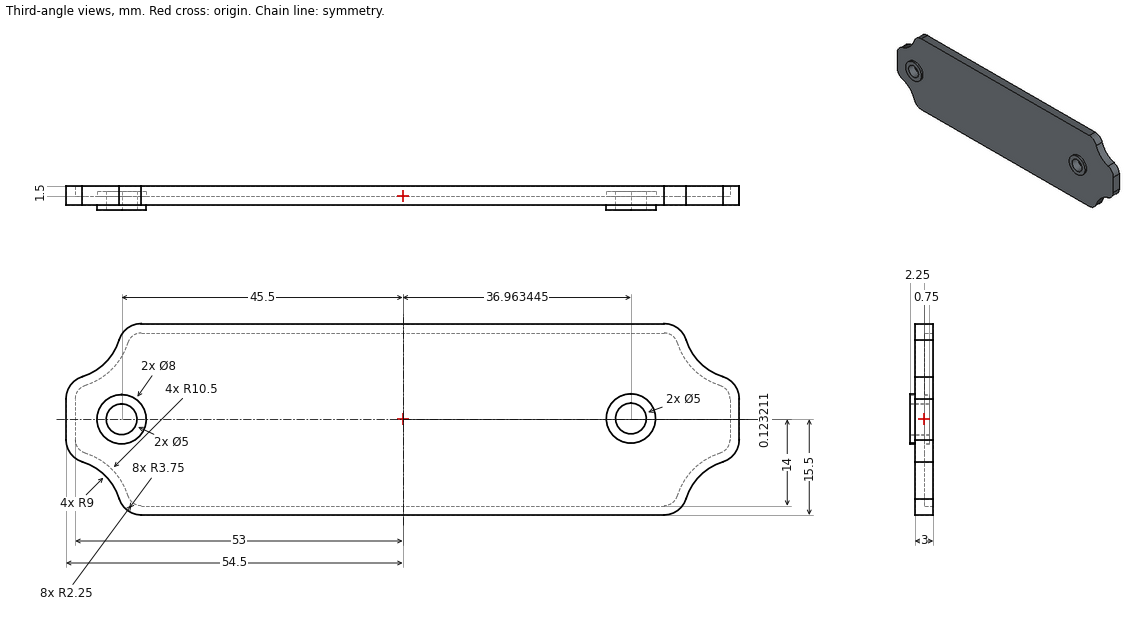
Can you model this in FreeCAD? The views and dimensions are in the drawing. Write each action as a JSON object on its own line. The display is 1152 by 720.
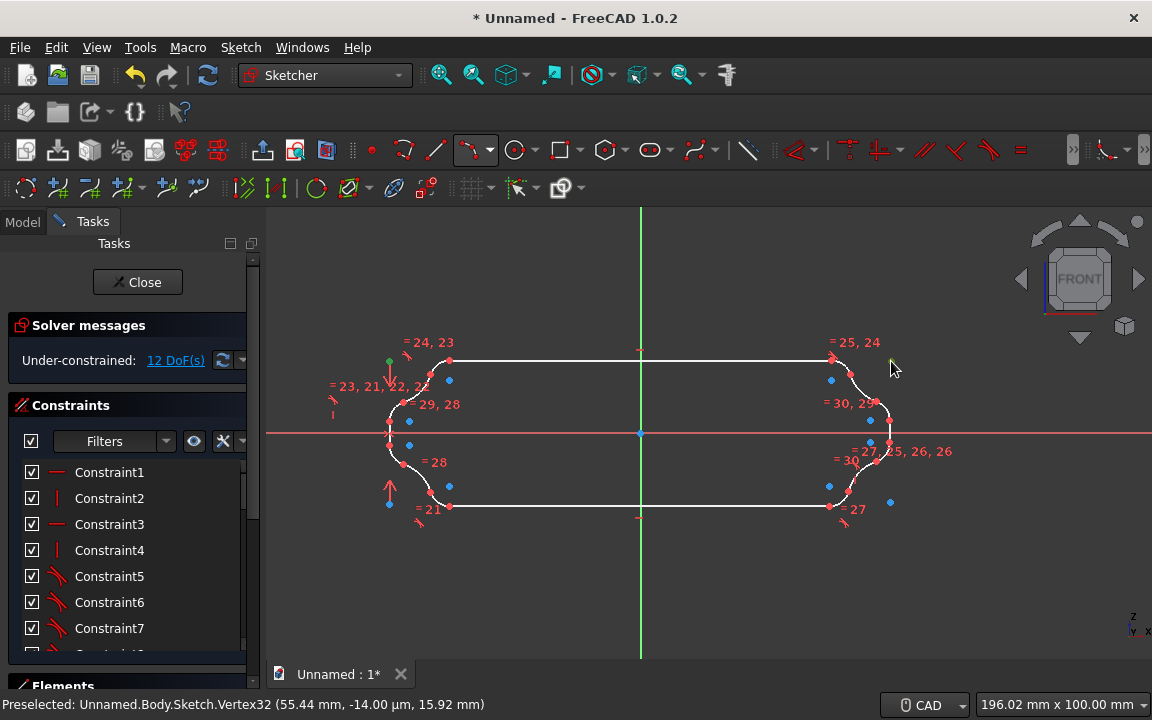
{"action": "left_click", "coordinate": [641, 603]}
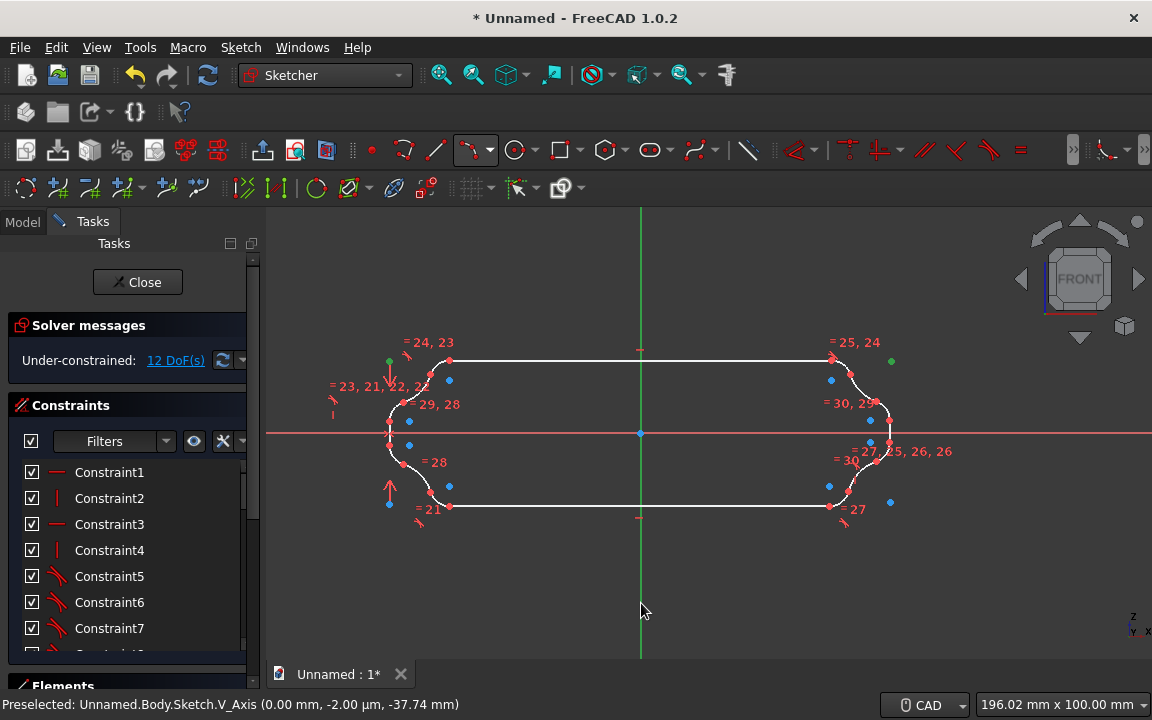
{"action": "key", "text": "s"}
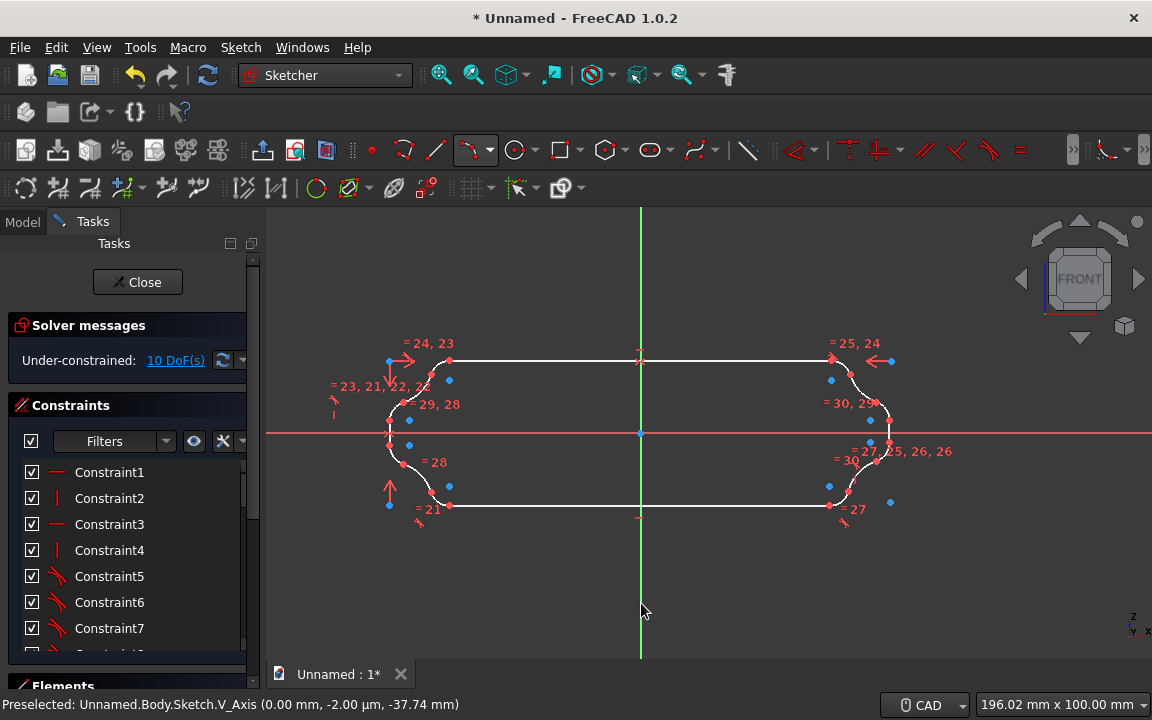
{"action": "left_click", "coordinate": [409, 446]}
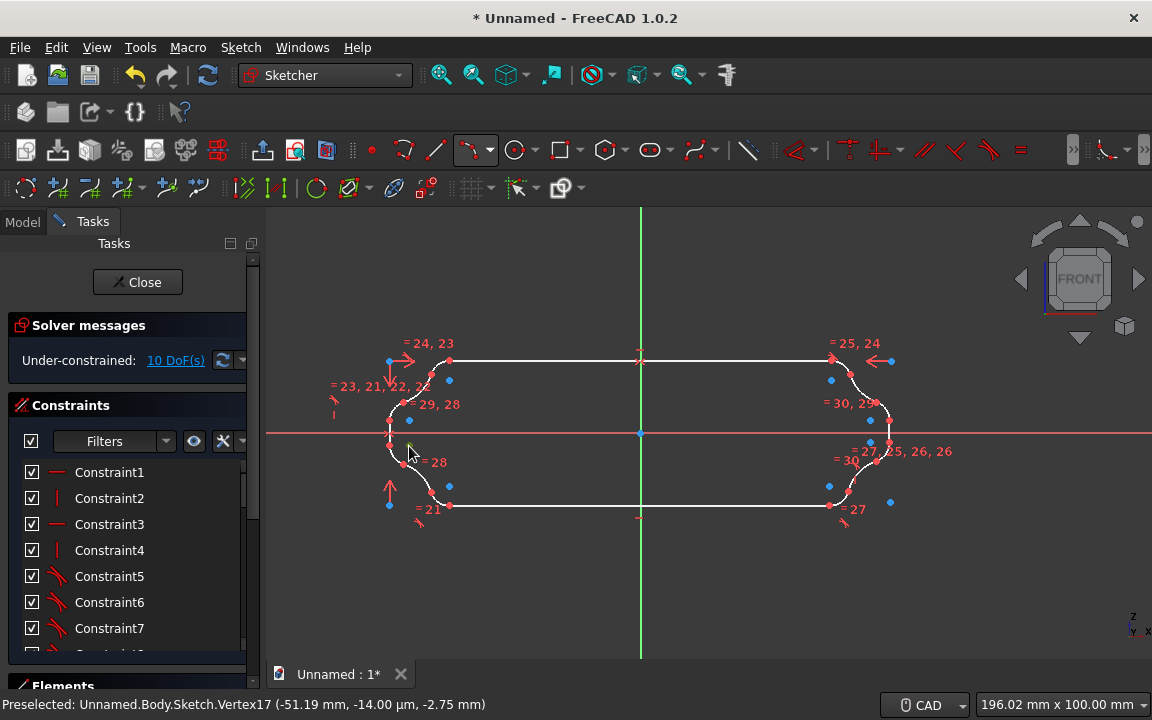
{"action": "left_click", "coordinate": [870, 443]}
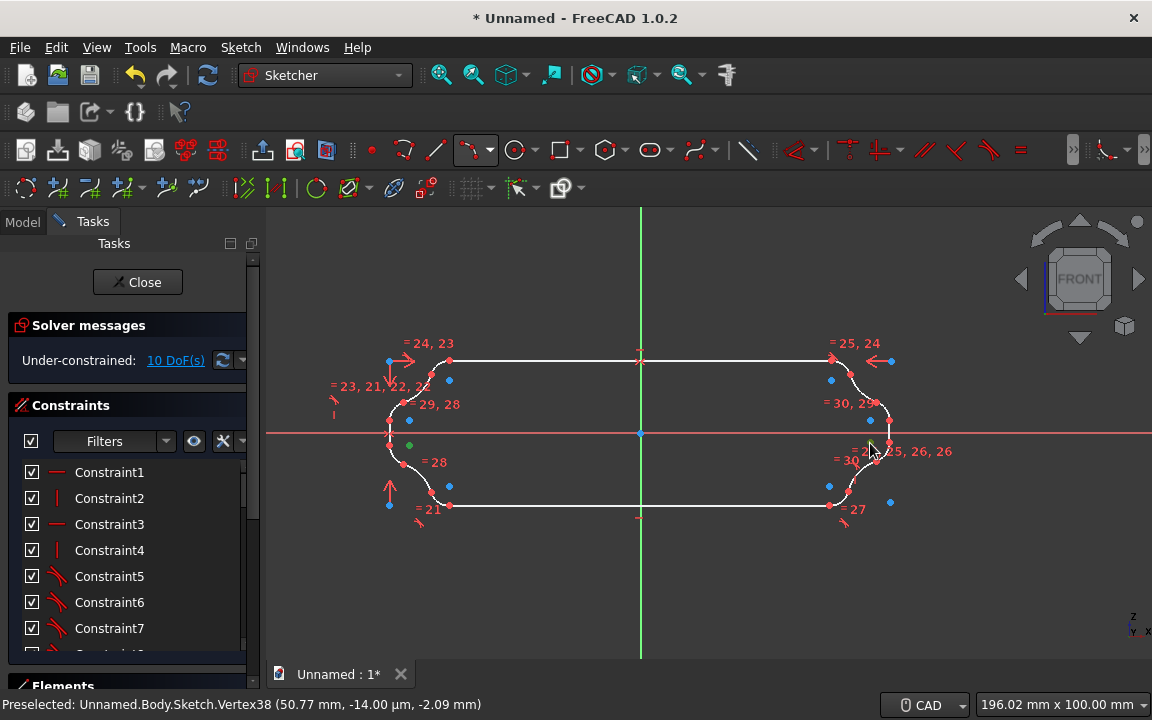
{"action": "left_click", "coordinate": [641, 603]}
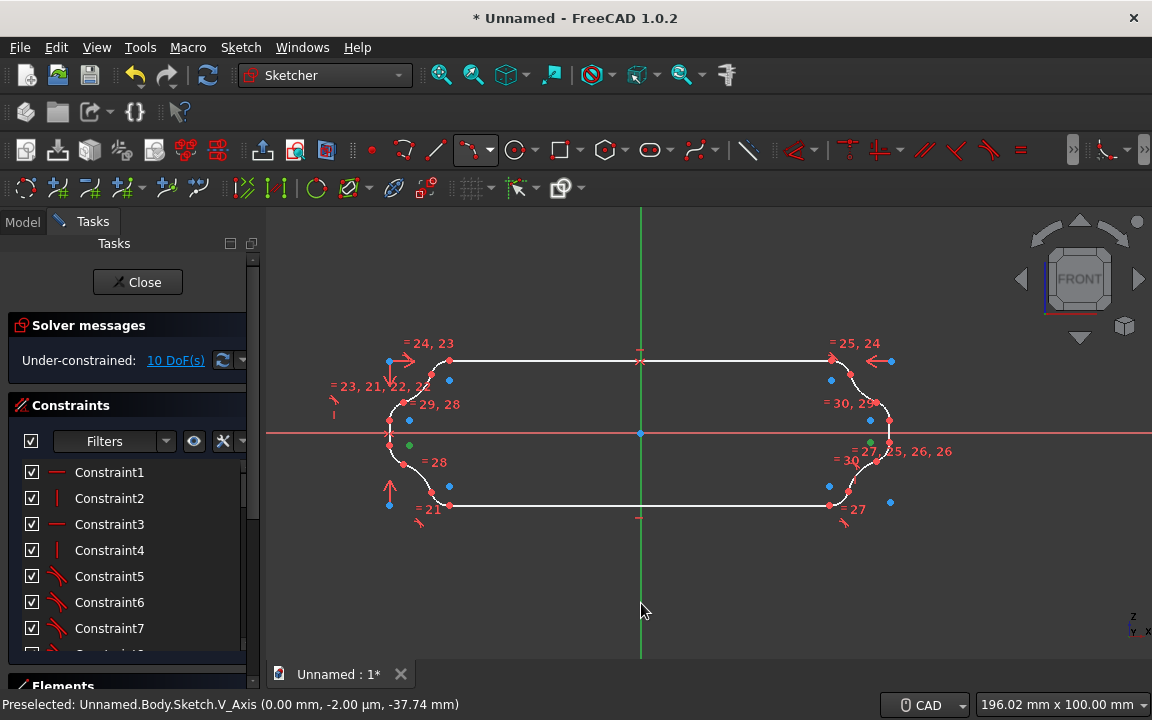
{"action": "key", "text": "s"}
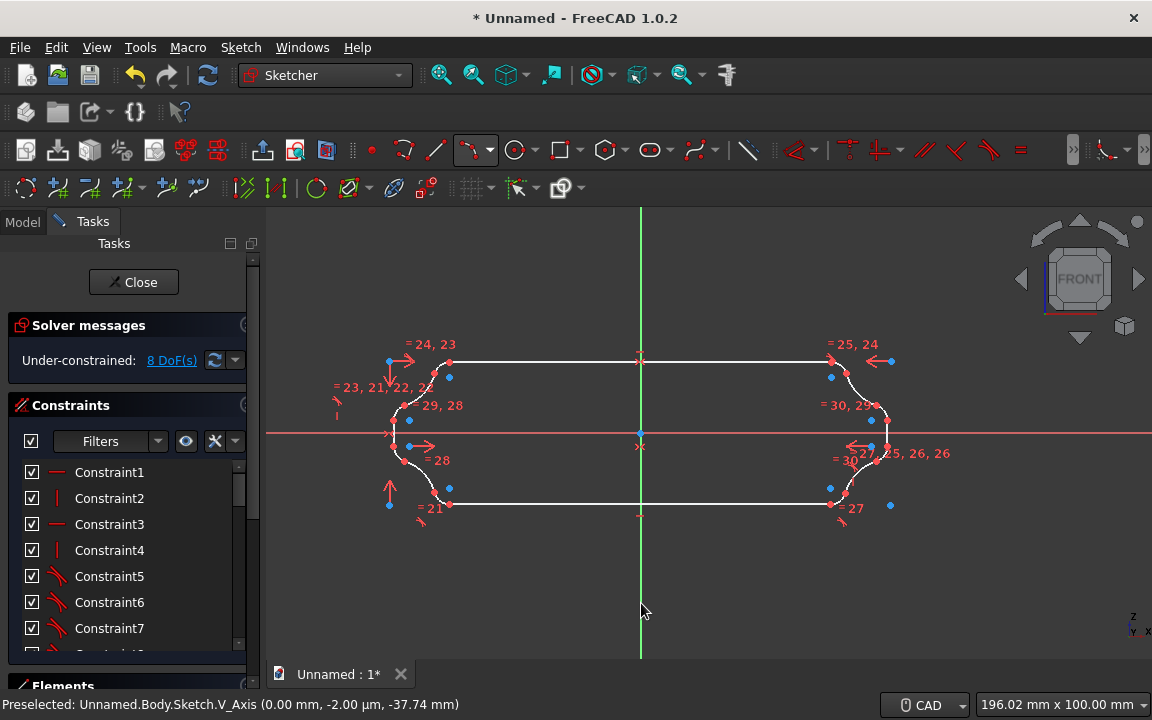
{"action": "left_click", "coordinate": [832, 378]}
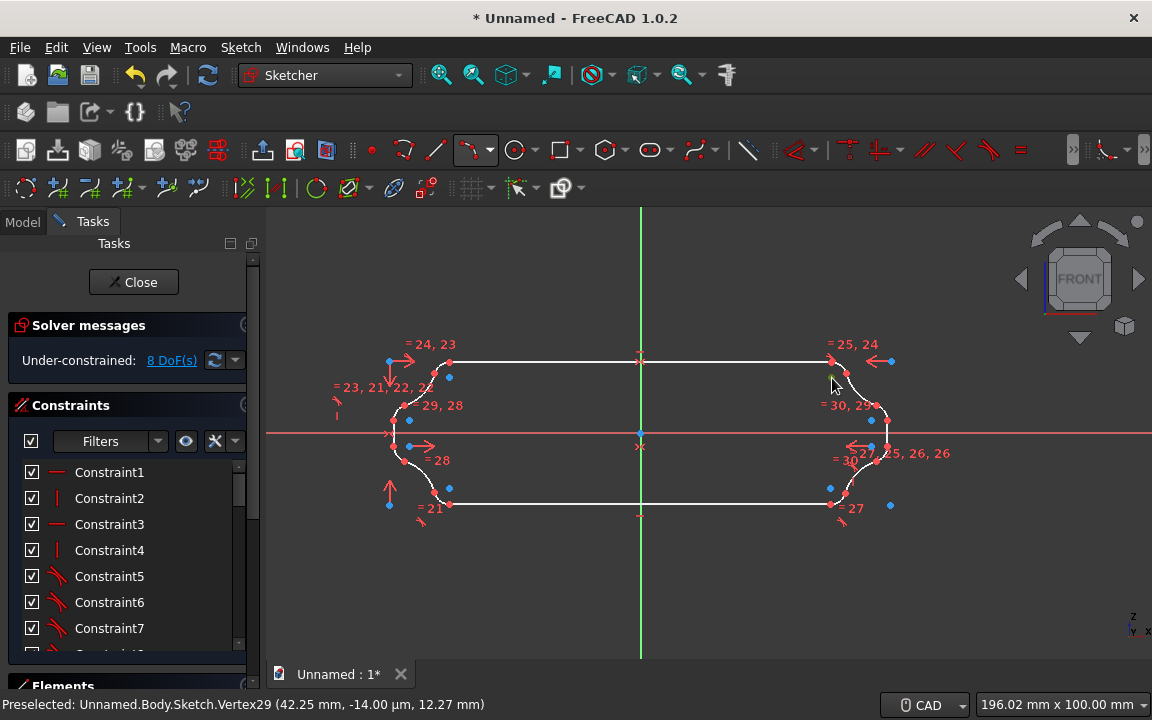
{"action": "left_click", "coordinate": [831, 489]}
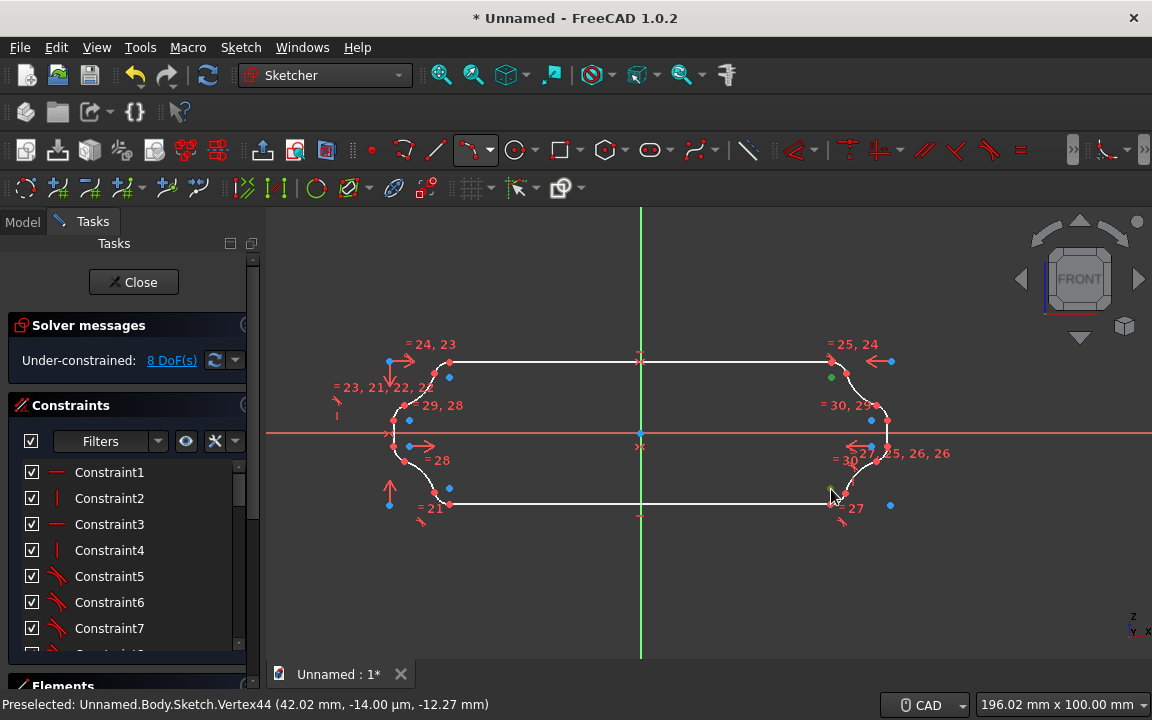
{"action": "left_click", "coordinate": [344, 433]}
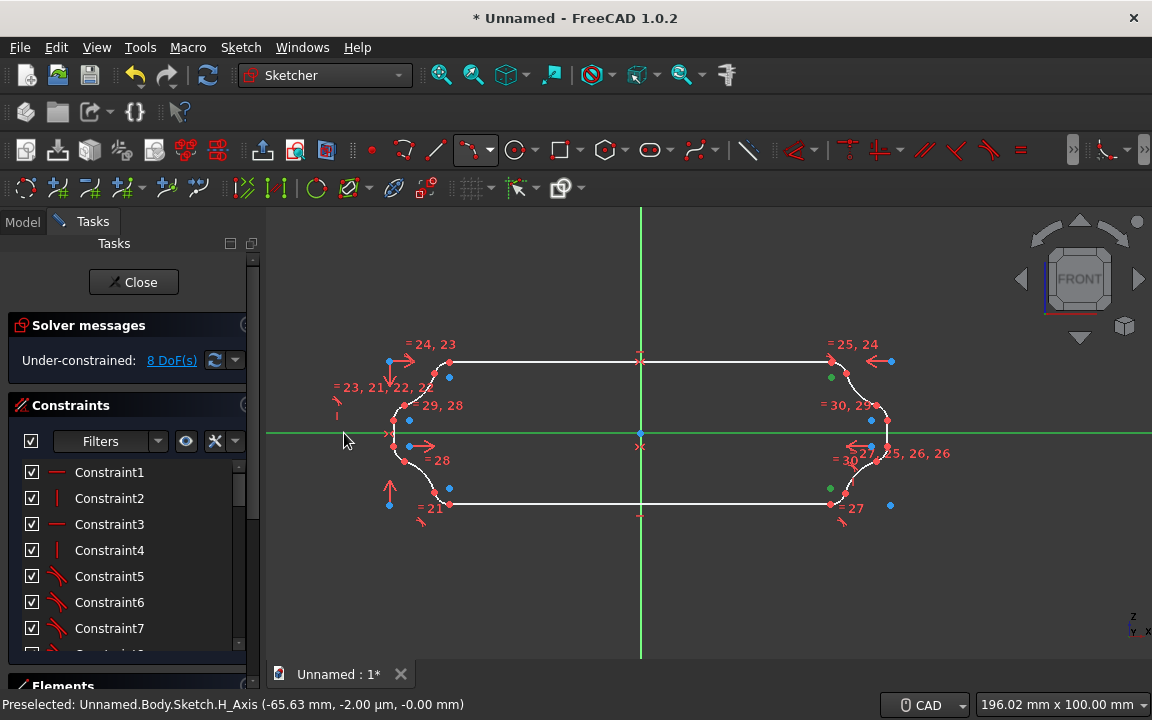
{"action": "key", "text": "s"}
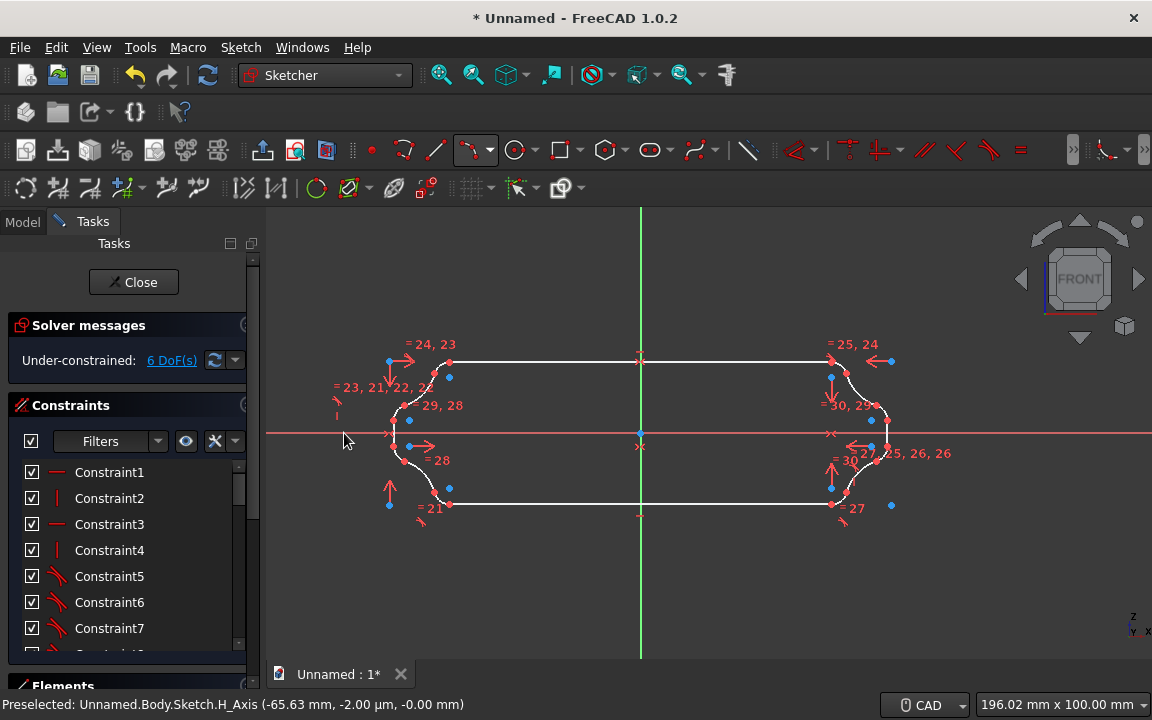
{"action": "scroll", "coordinate": [440, 501], "scroll_direction": "up", "scroll_amount": 5}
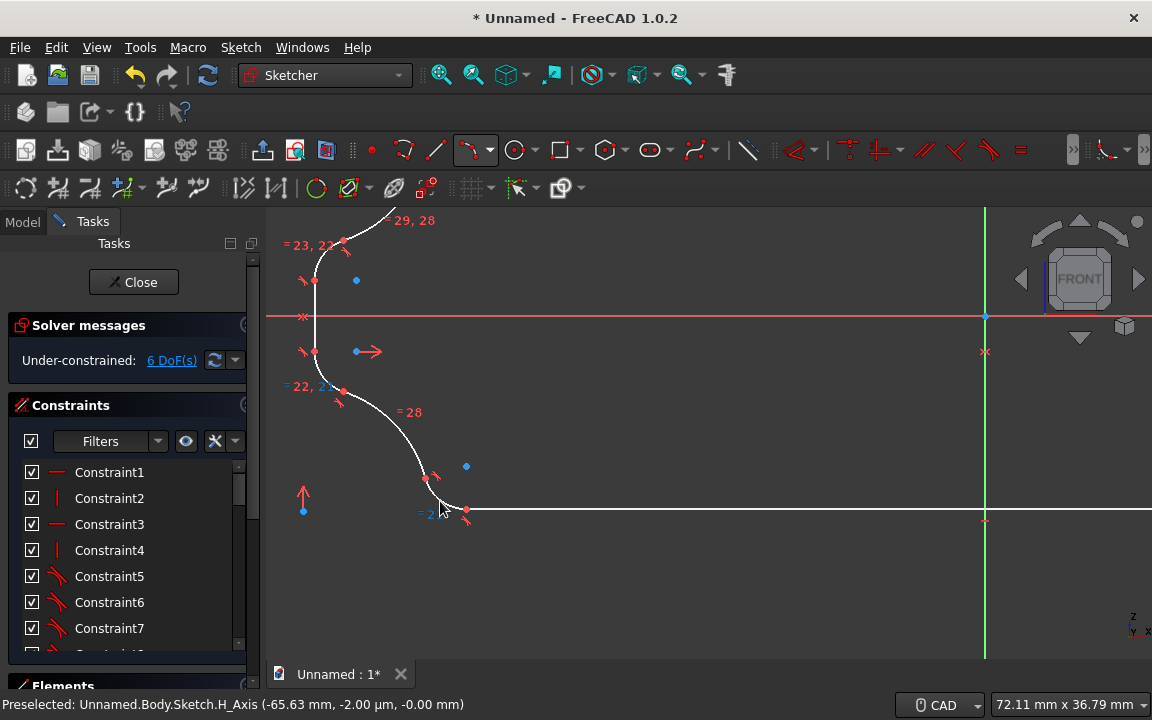
{"action": "left_click", "coordinate": [441, 500]}